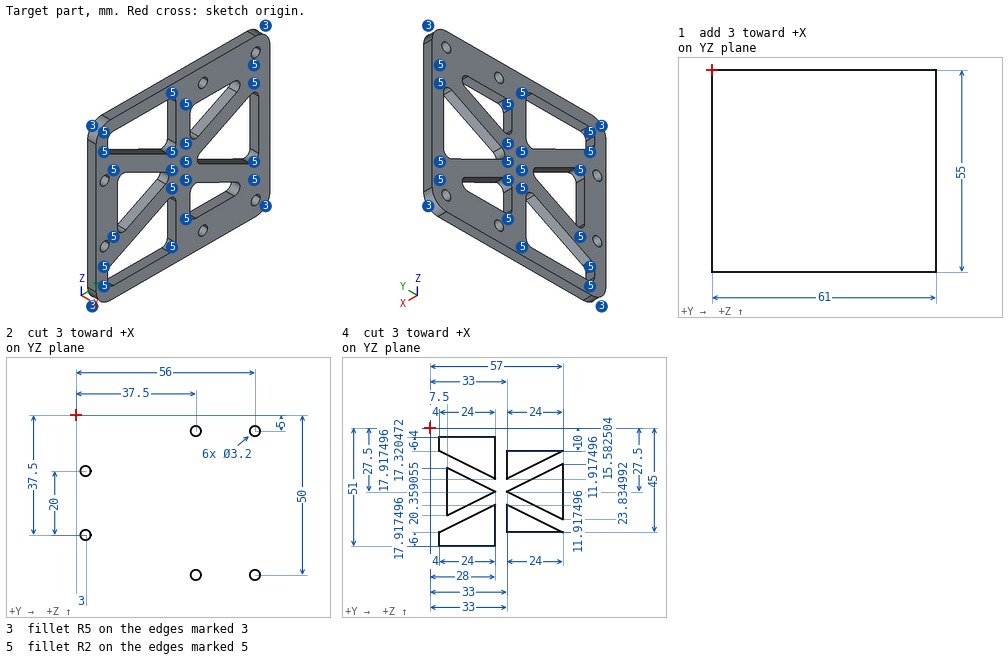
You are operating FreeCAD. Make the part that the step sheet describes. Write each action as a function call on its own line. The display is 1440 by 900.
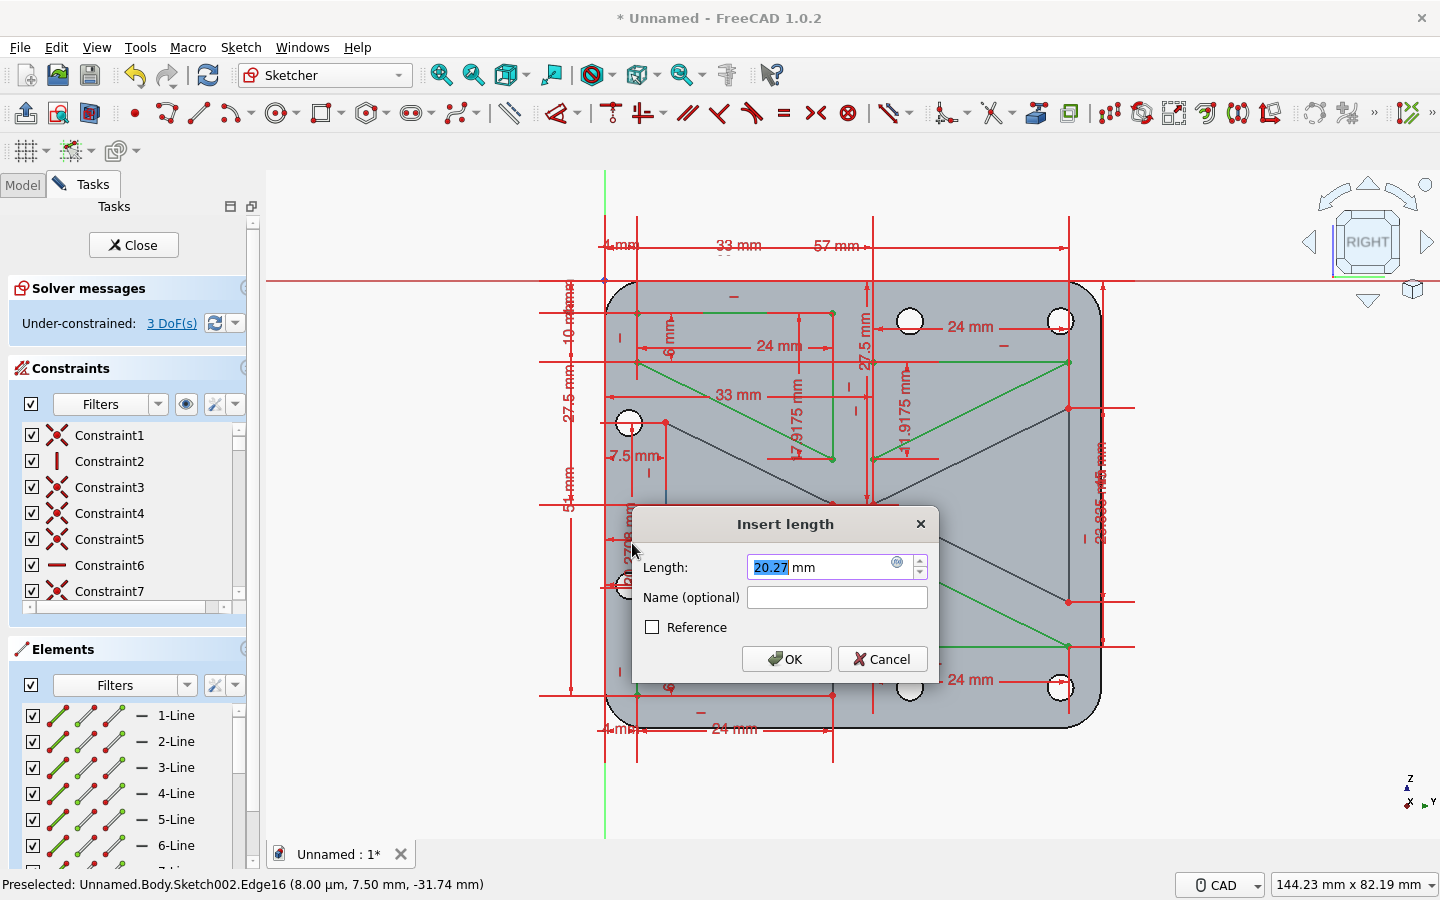
text(20.359055)
key(Return)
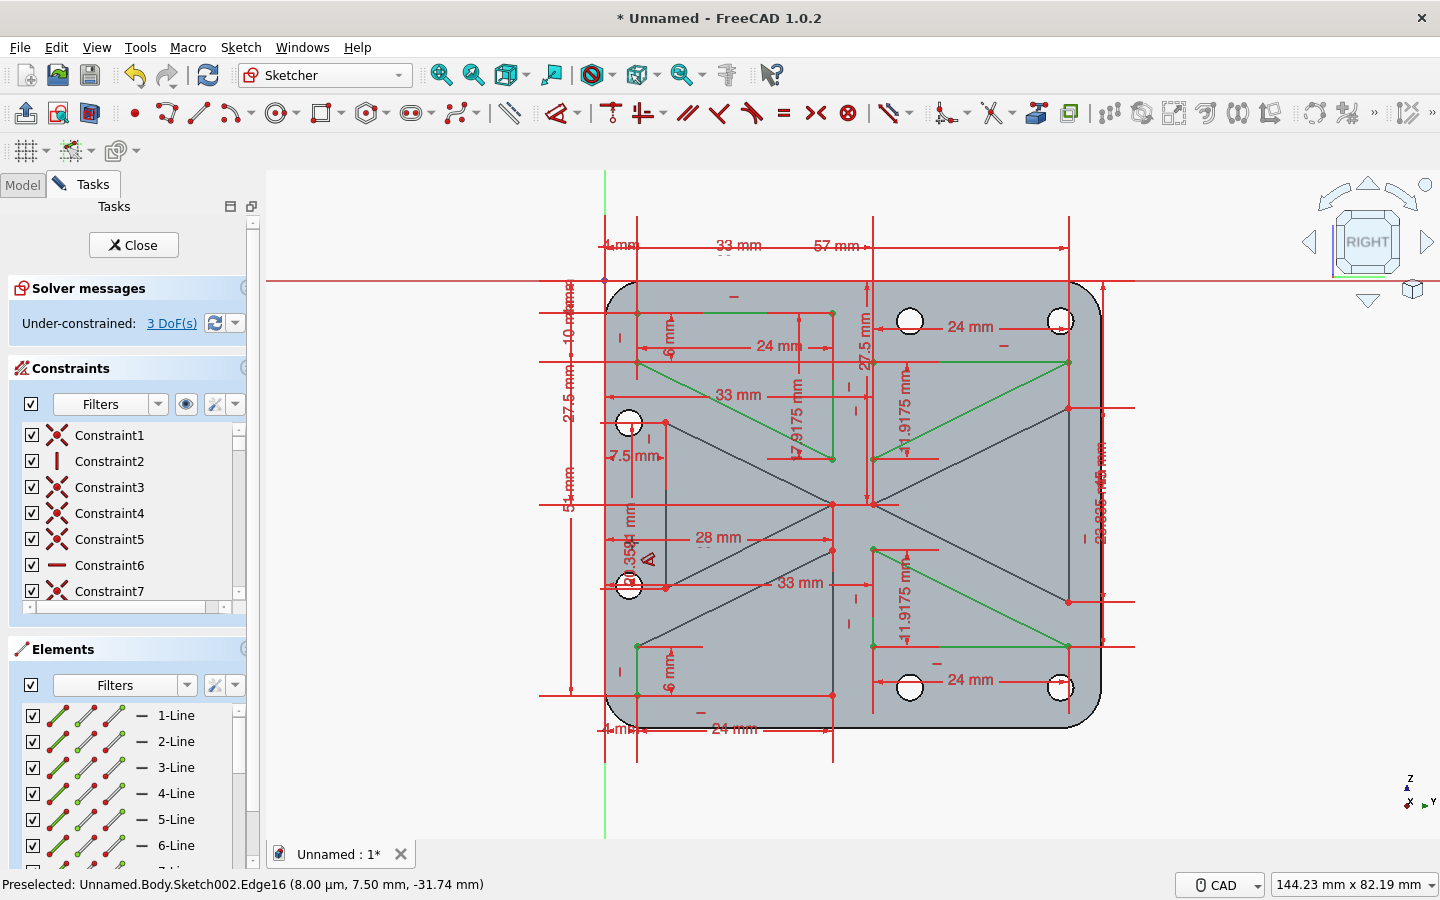
click(833, 594)
click(799, 623)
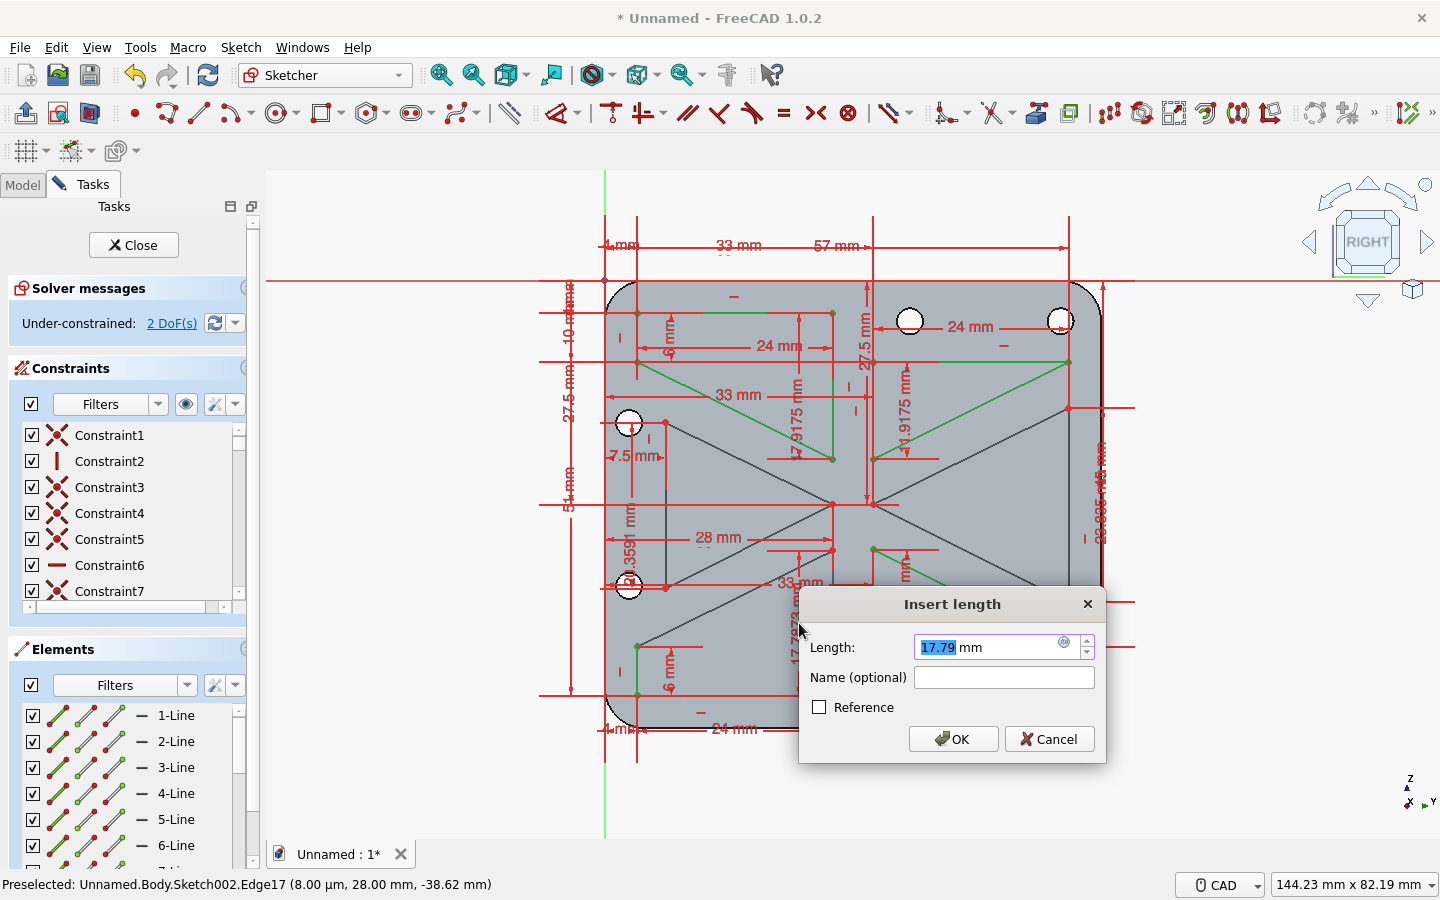
text(17.917496)
key(Return)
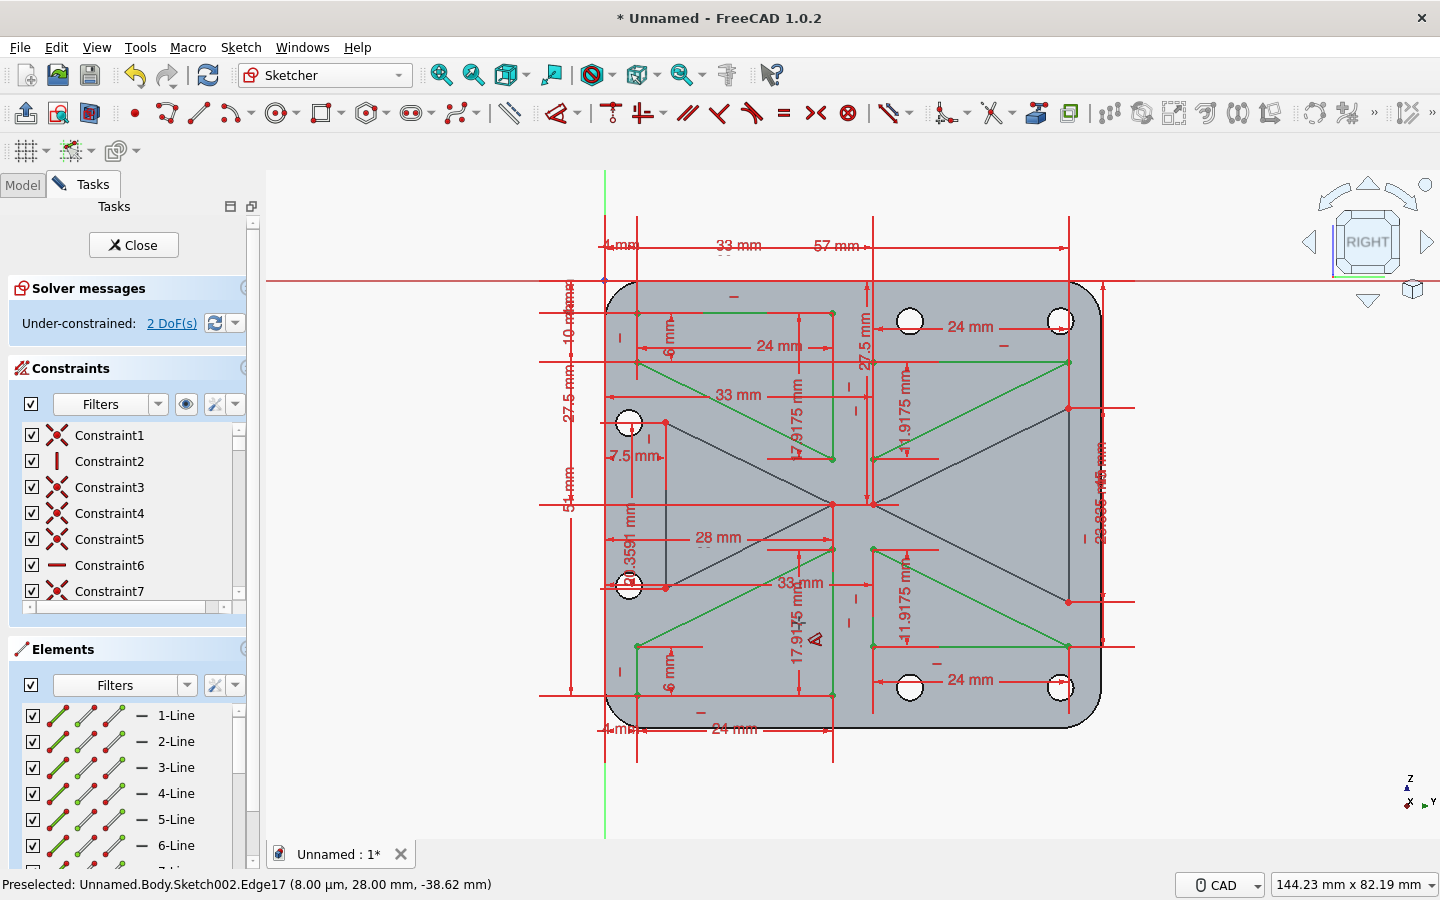
click(1069, 408)
click(1103, 344)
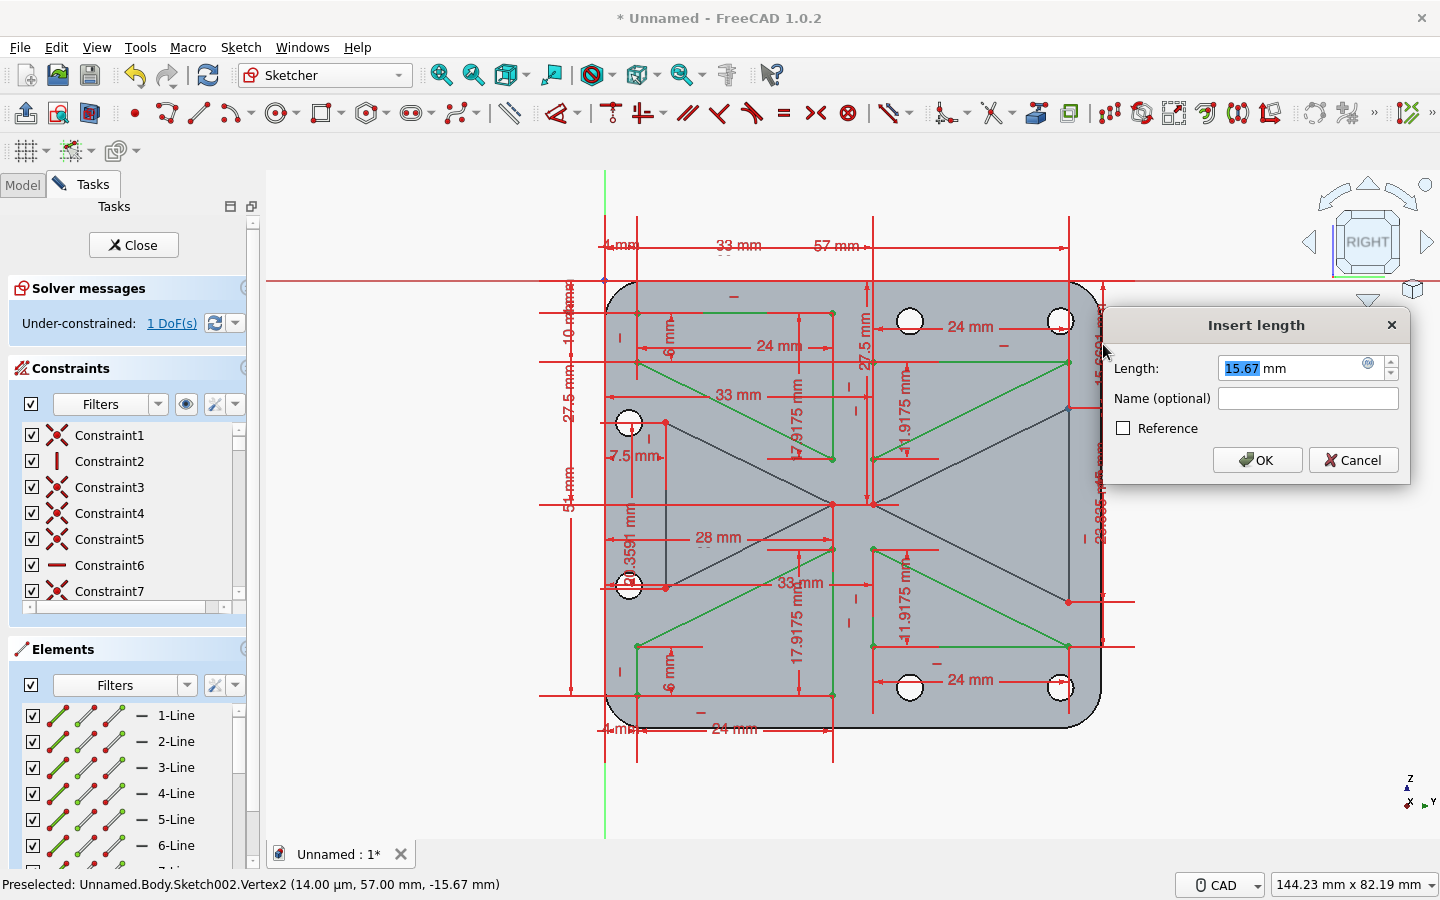
text(15.582504)
key(Return)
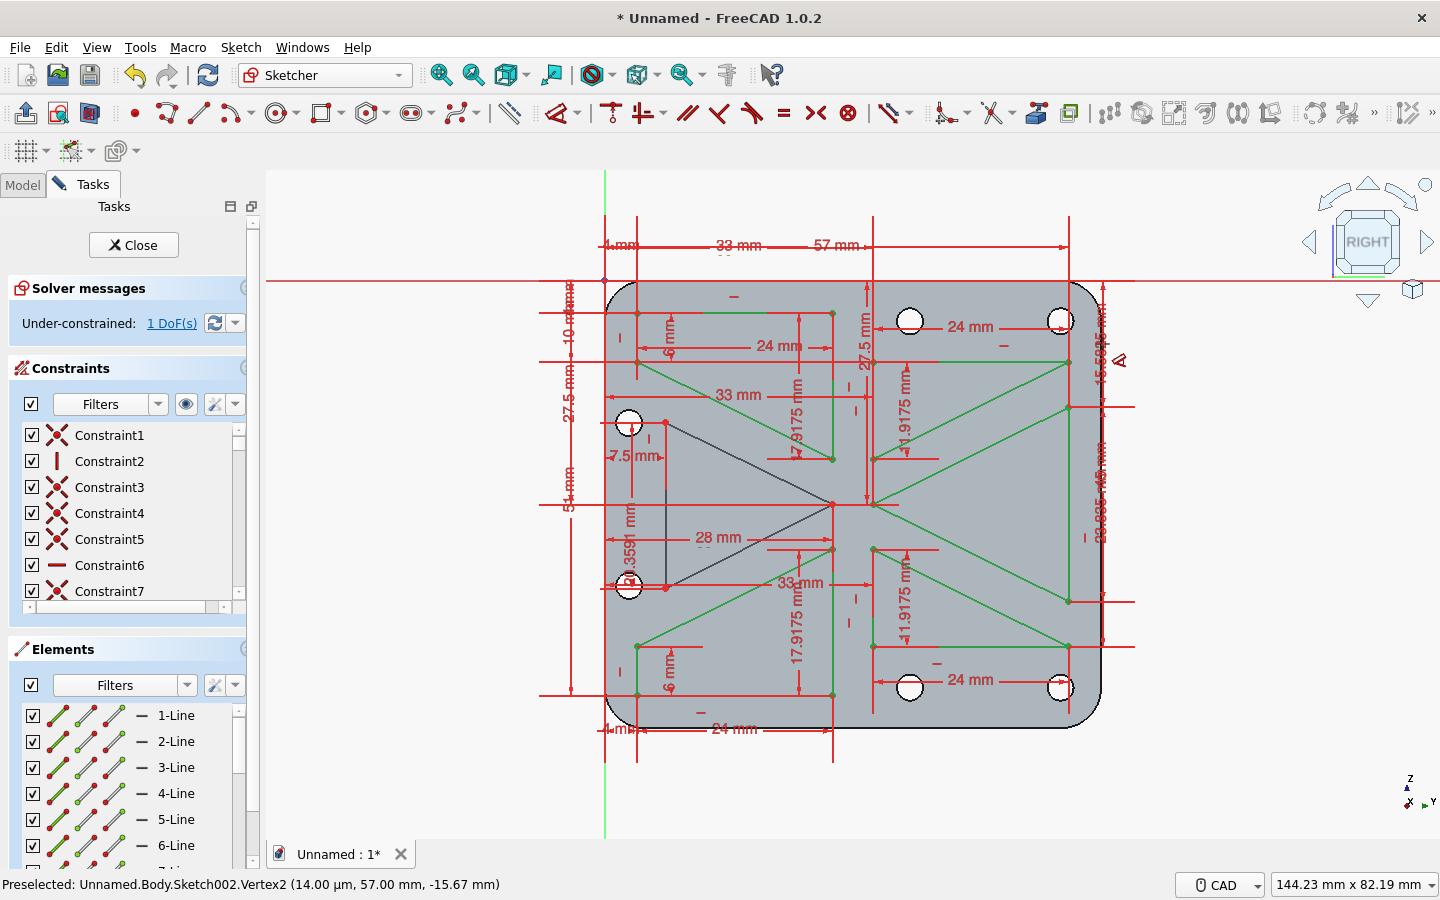
click(666, 423)
click(571, 352)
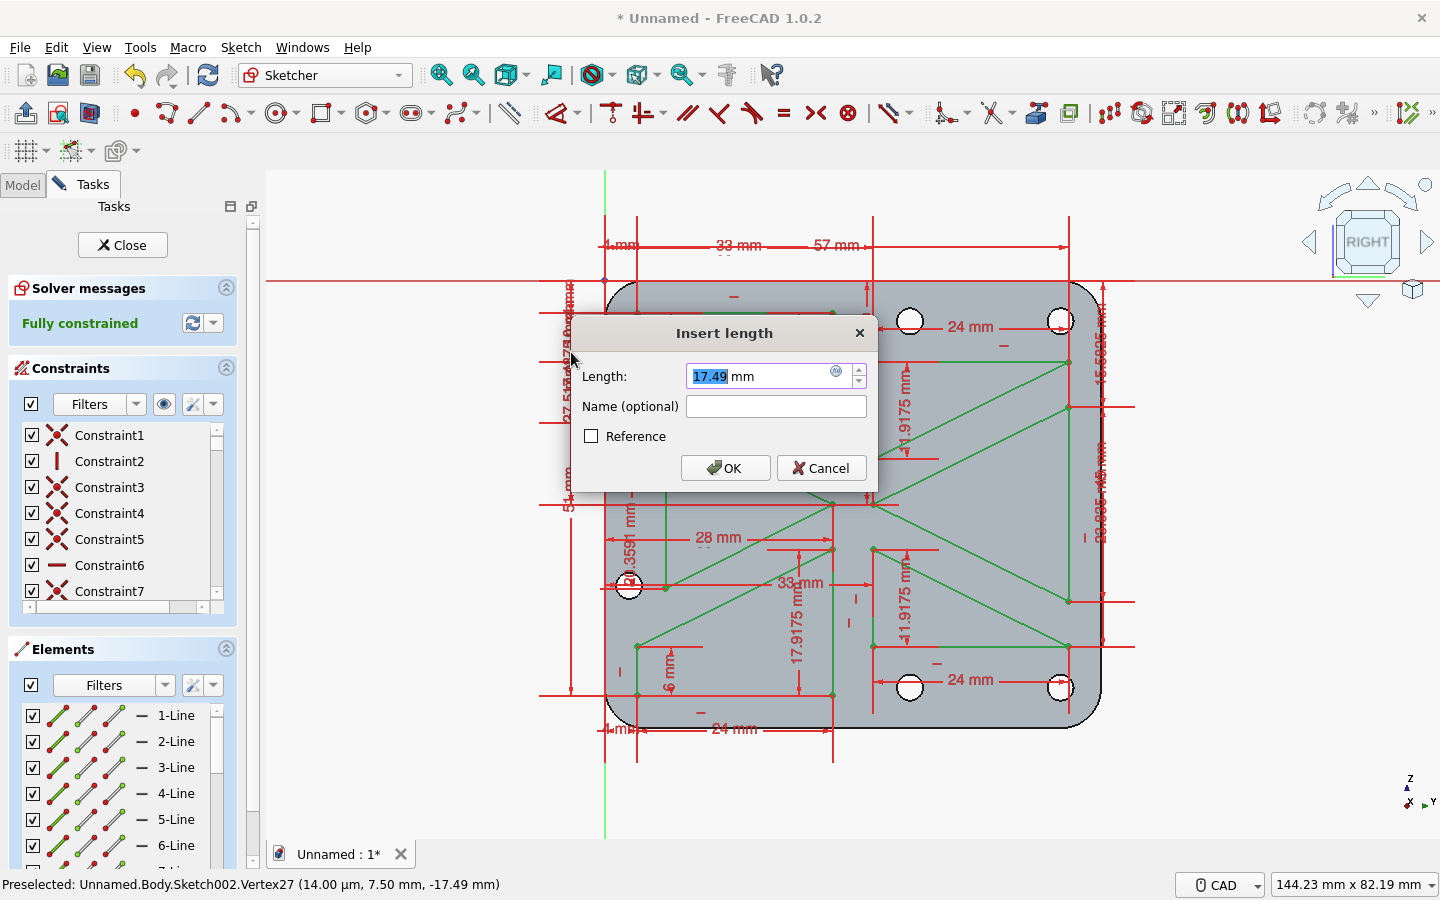
text(17.320472)
key(Return)
key(Escape)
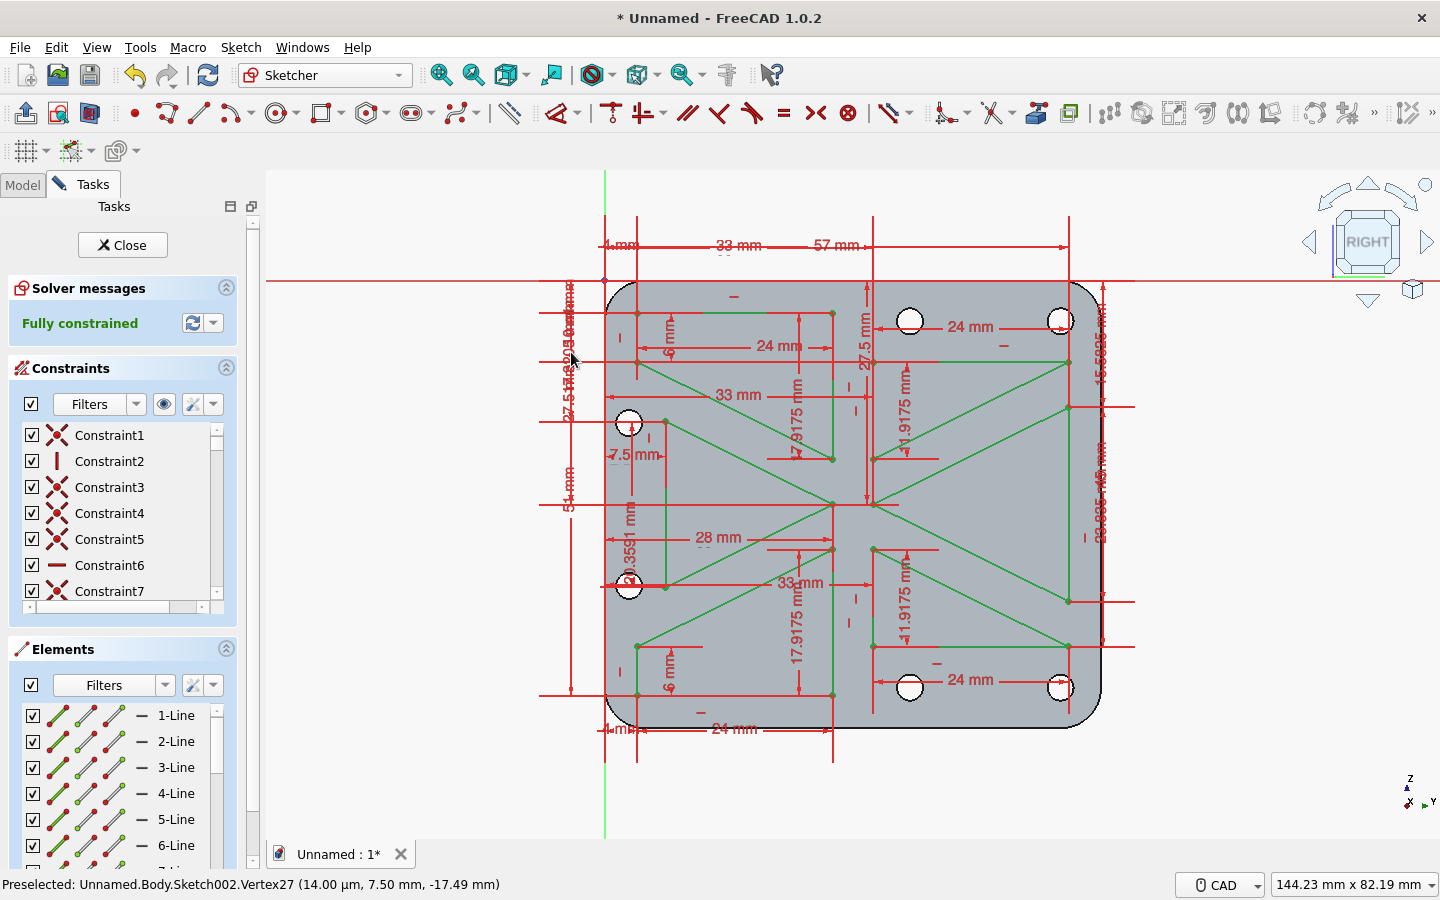
click(123, 245)